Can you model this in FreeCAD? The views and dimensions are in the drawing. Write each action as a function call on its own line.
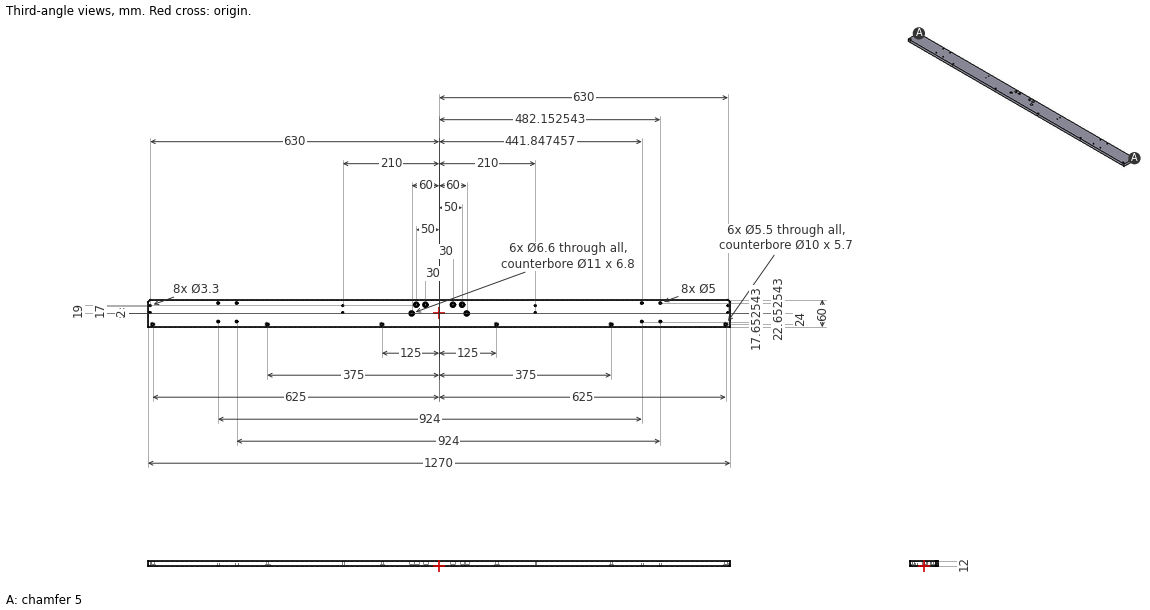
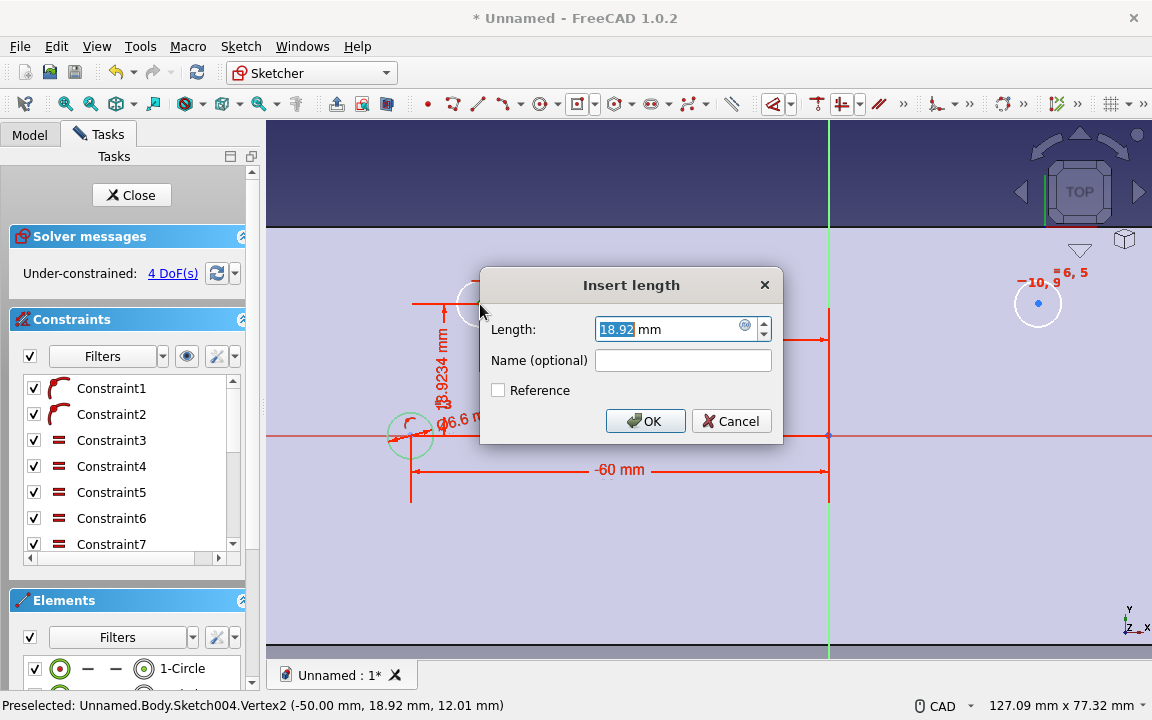
text(19)
key(Return)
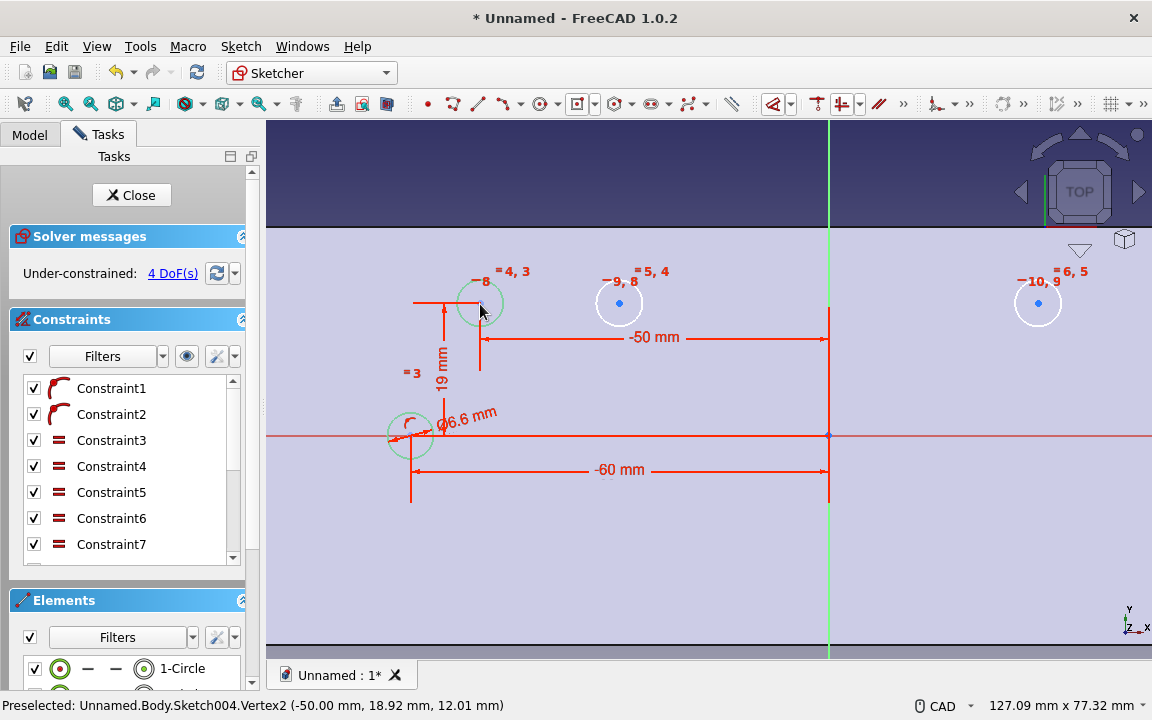
click(619, 303)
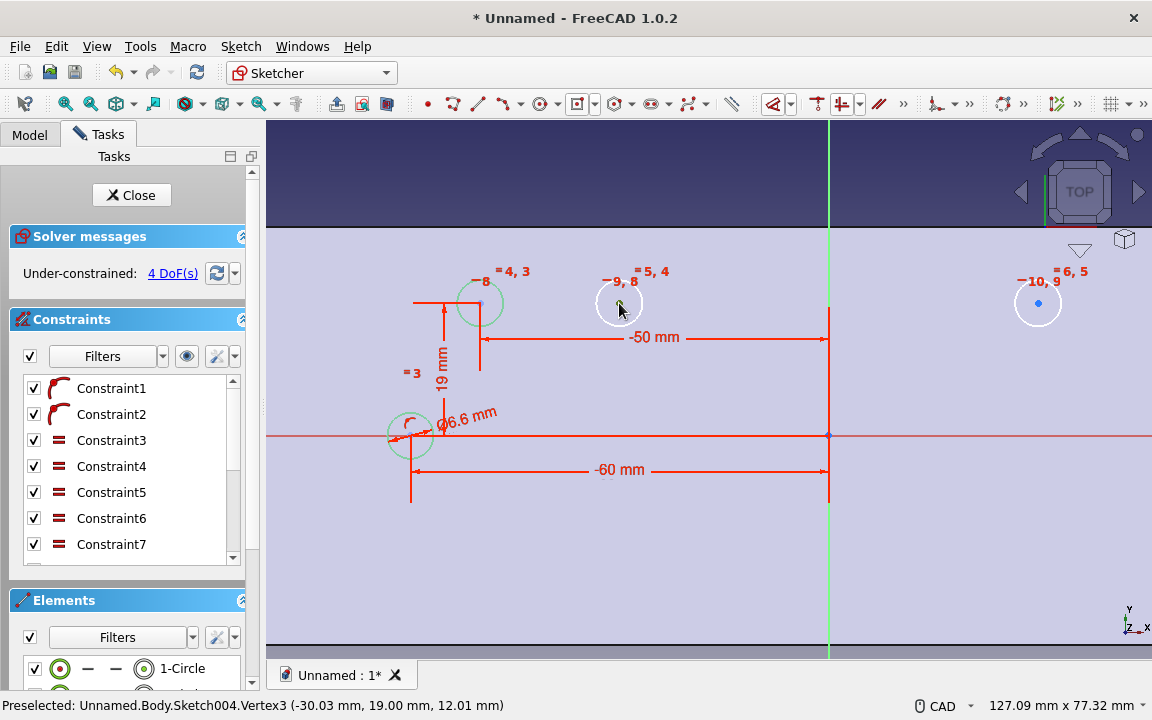
click(790, 104)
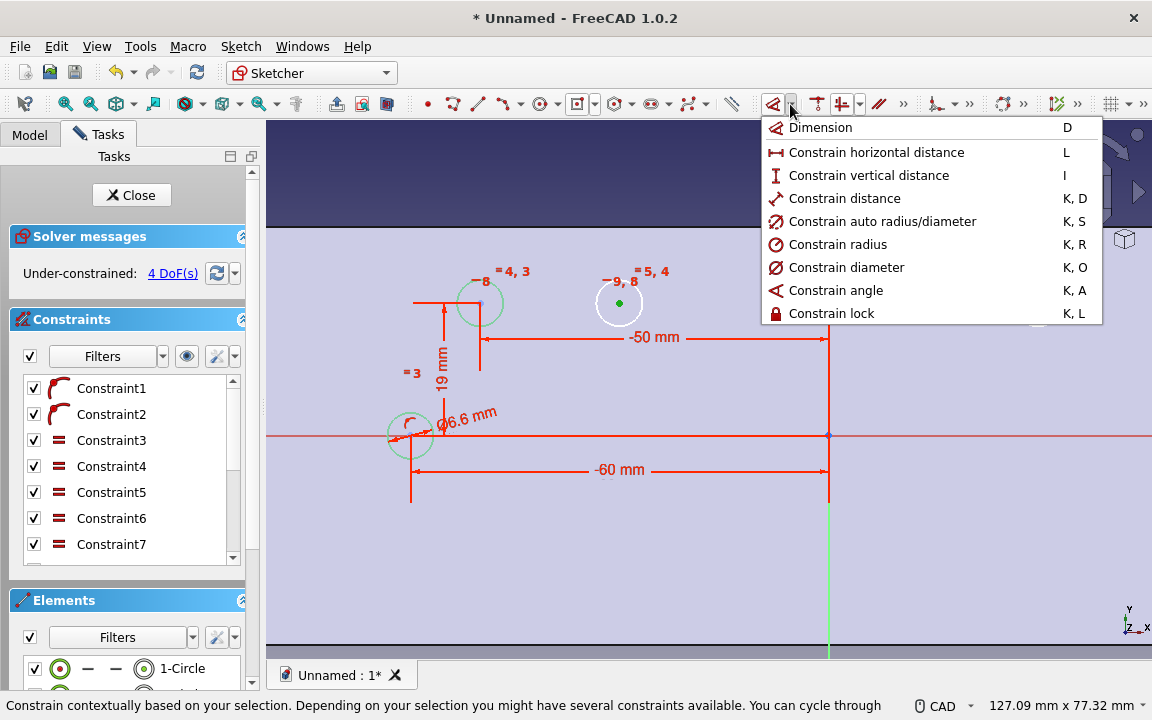
click(932, 152)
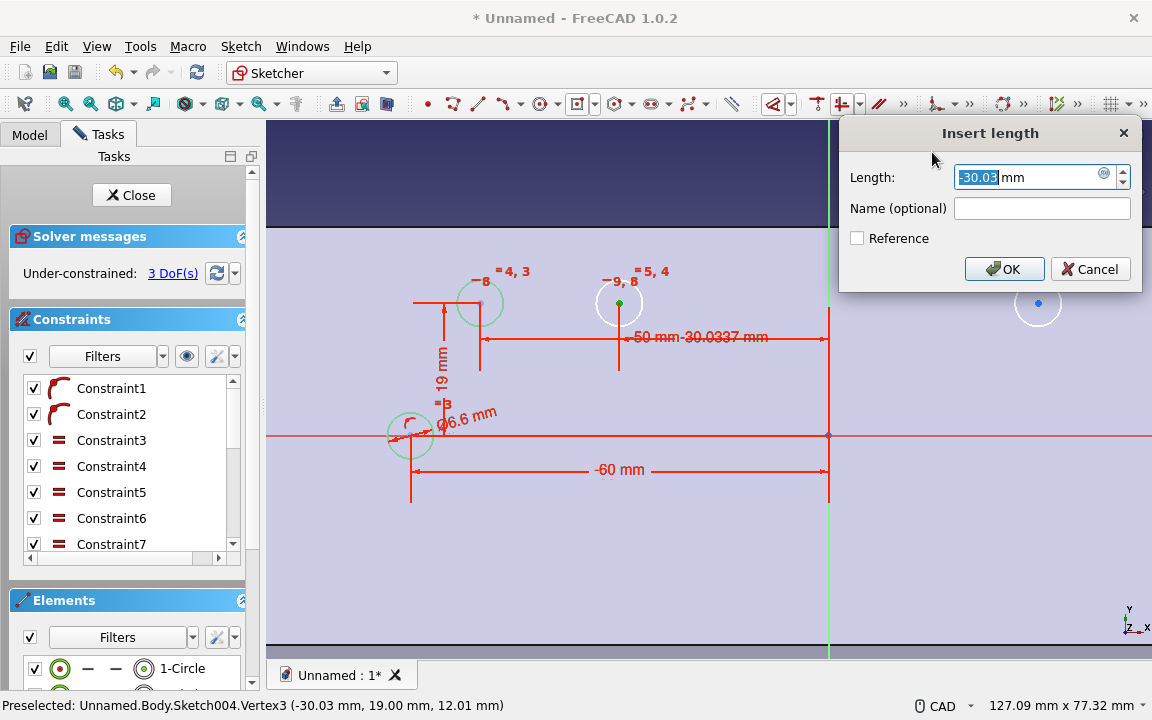
text(-30)
key(Return)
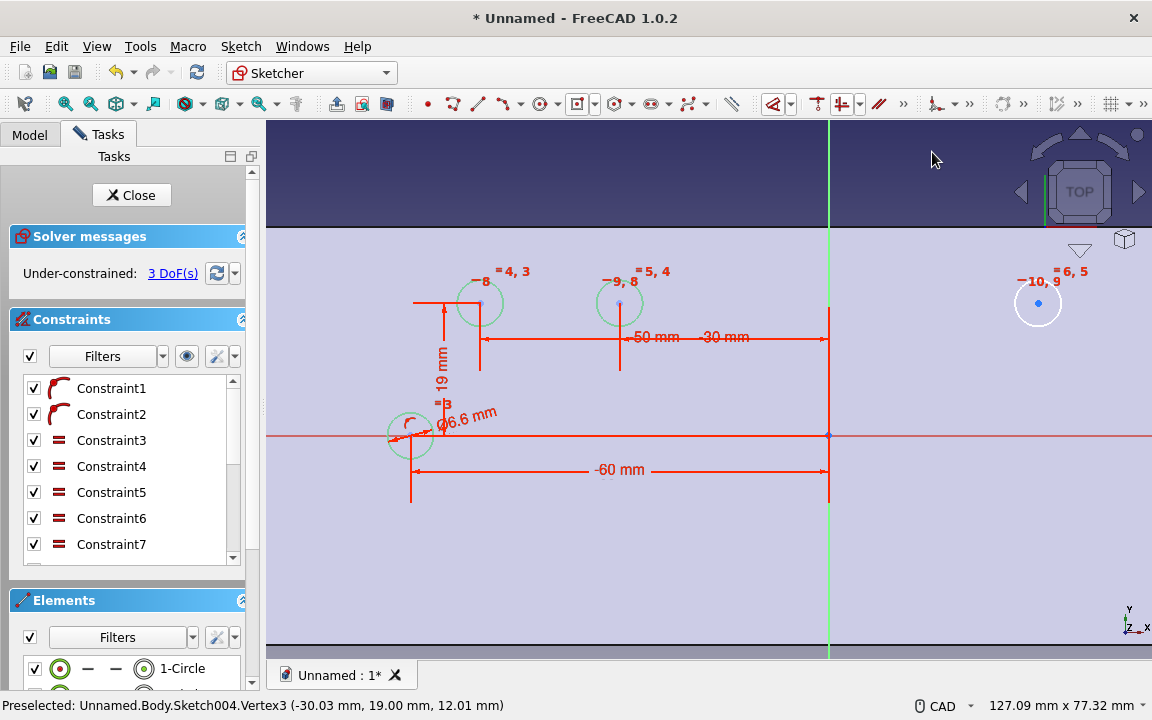
scroll(411, 414, down, 3)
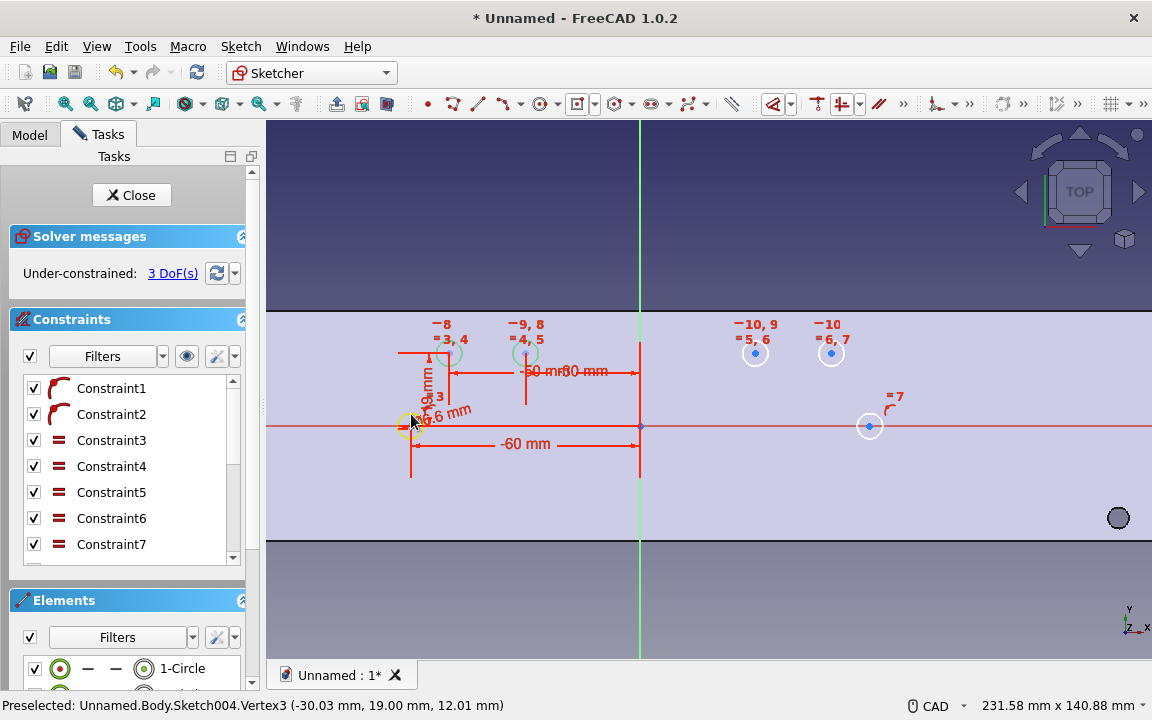
click(755, 353)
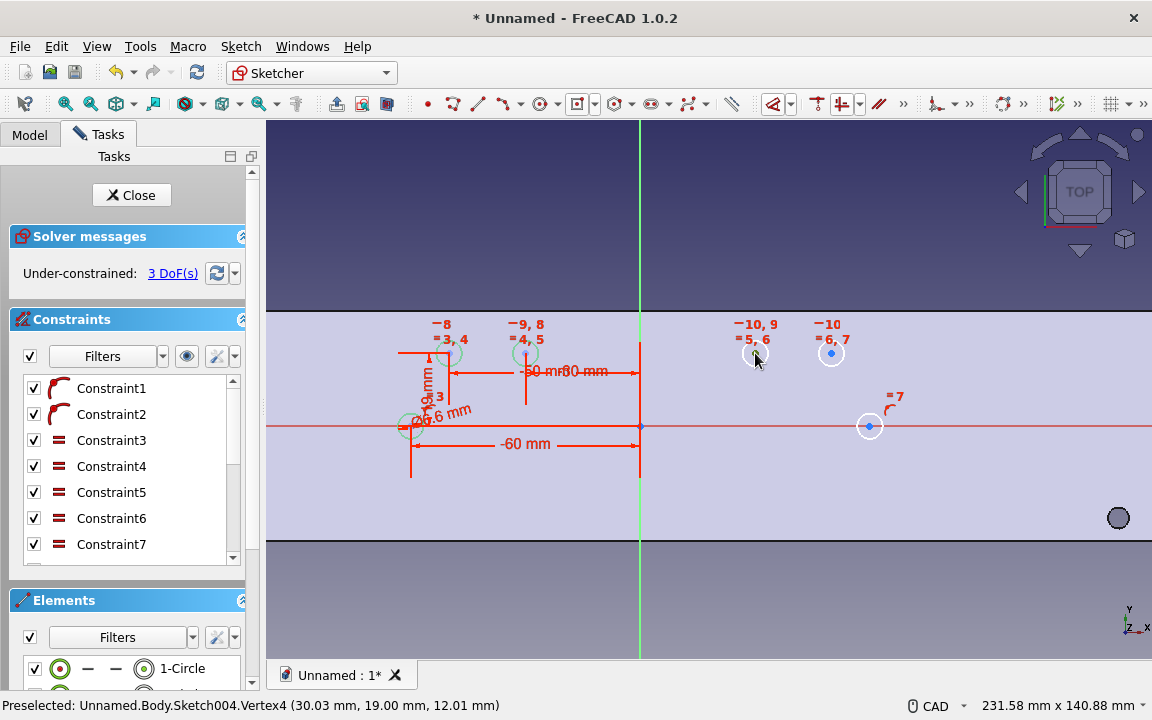
key(l)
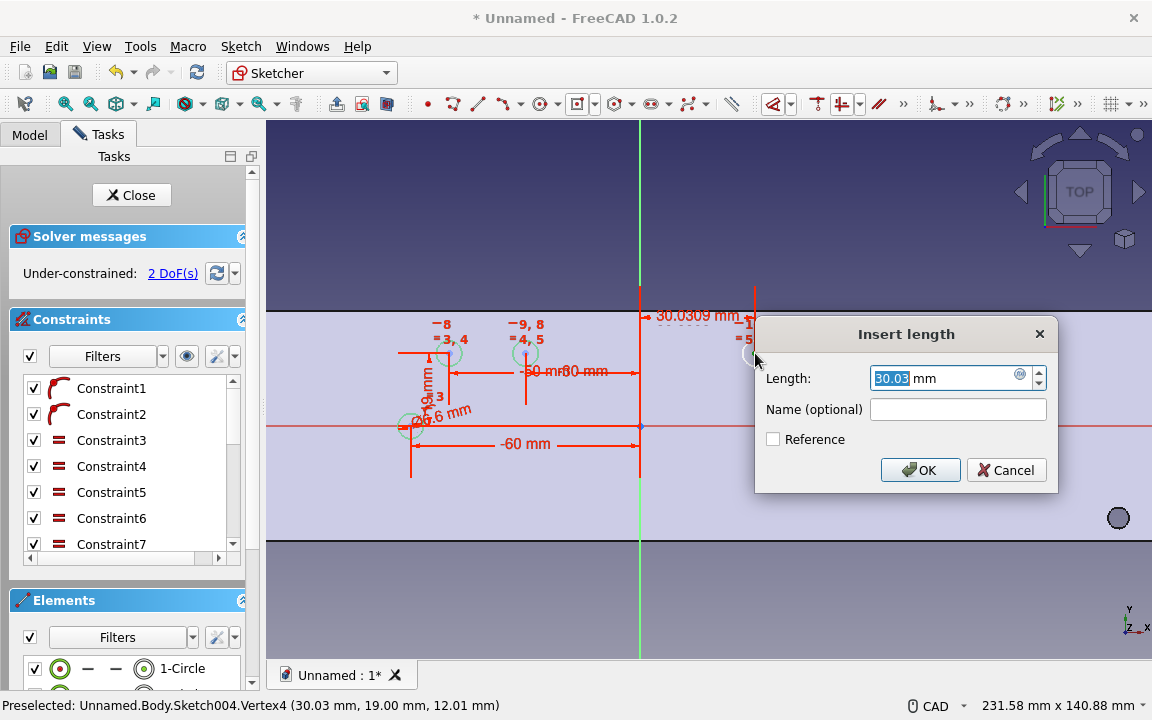
text(30)
key(Return)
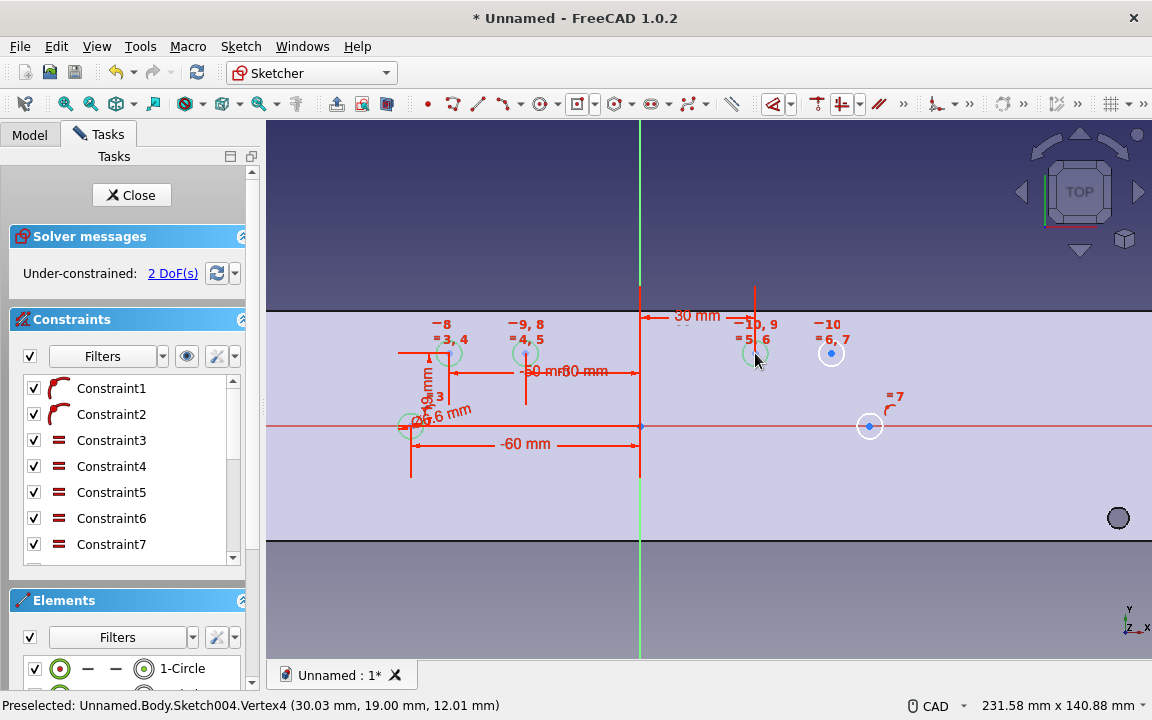
click(832, 353)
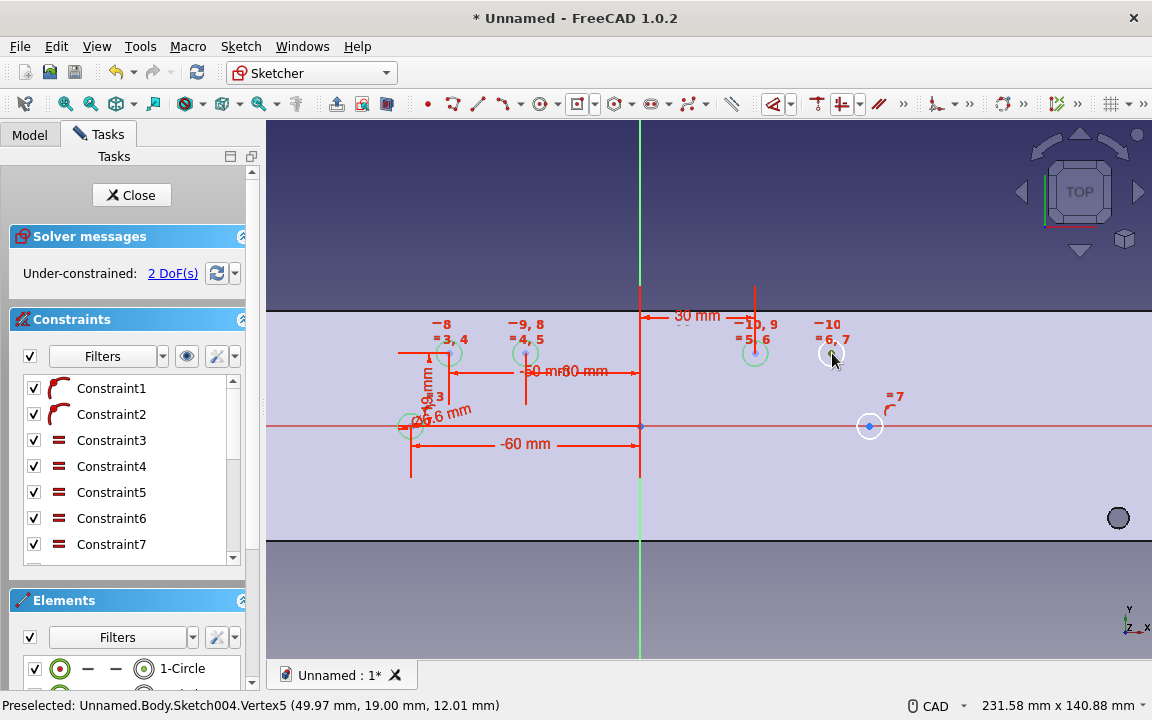
click(790, 104)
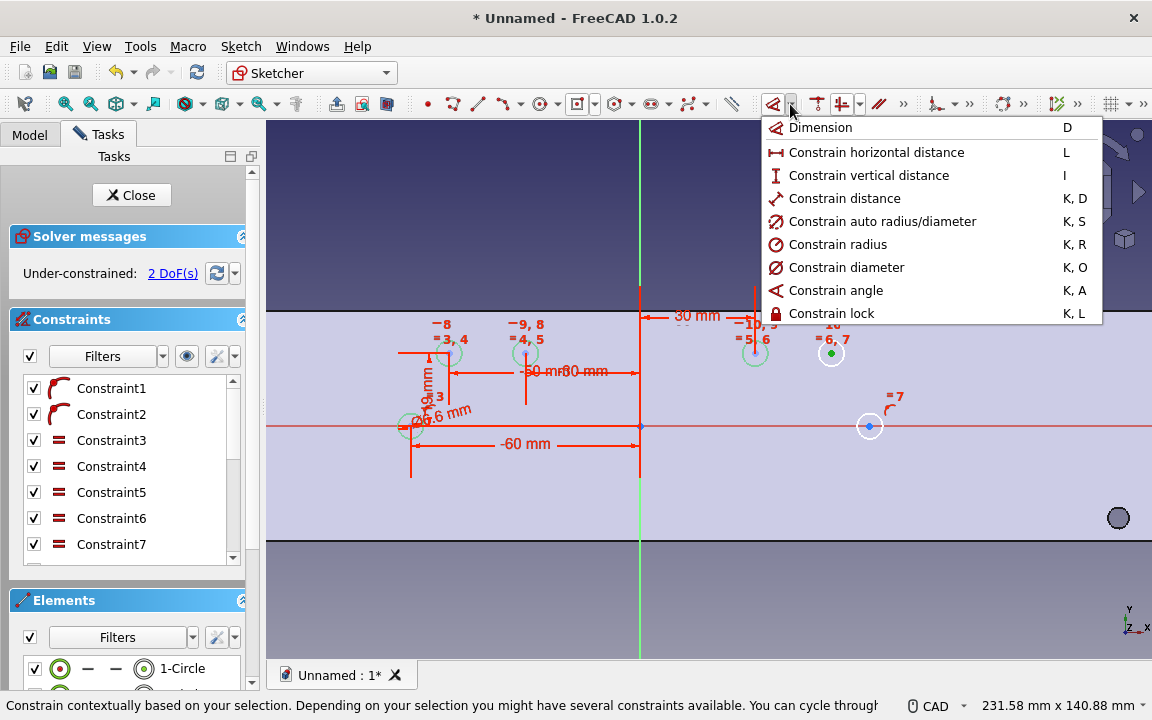
click(932, 152)